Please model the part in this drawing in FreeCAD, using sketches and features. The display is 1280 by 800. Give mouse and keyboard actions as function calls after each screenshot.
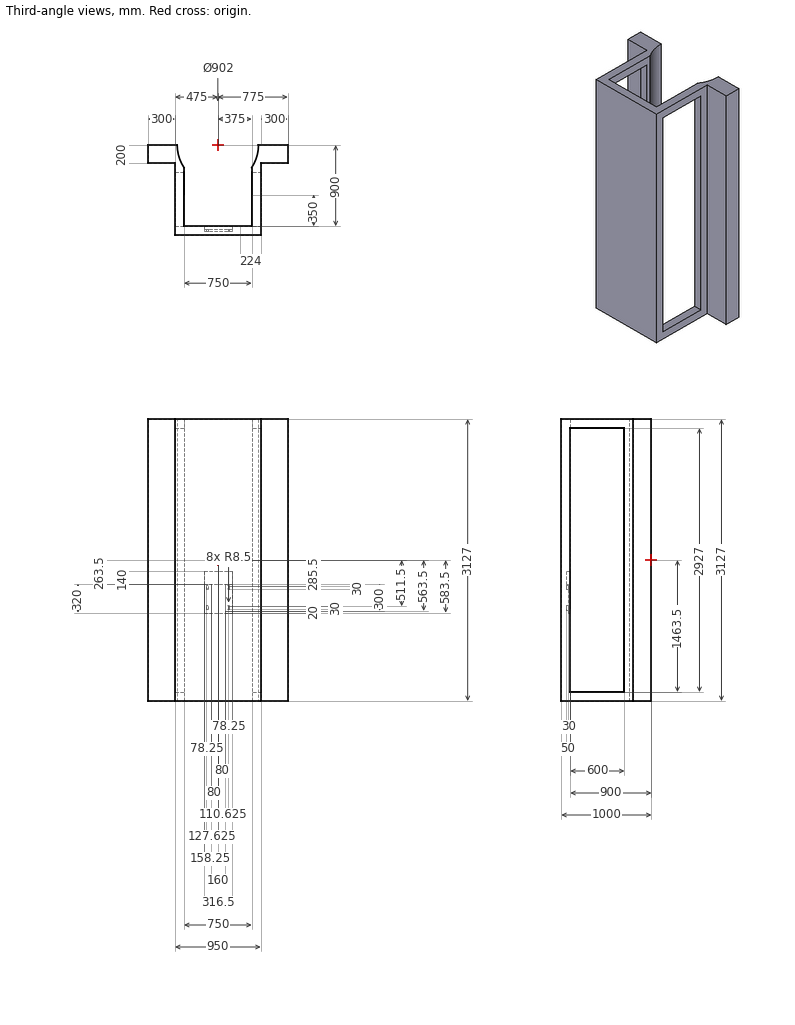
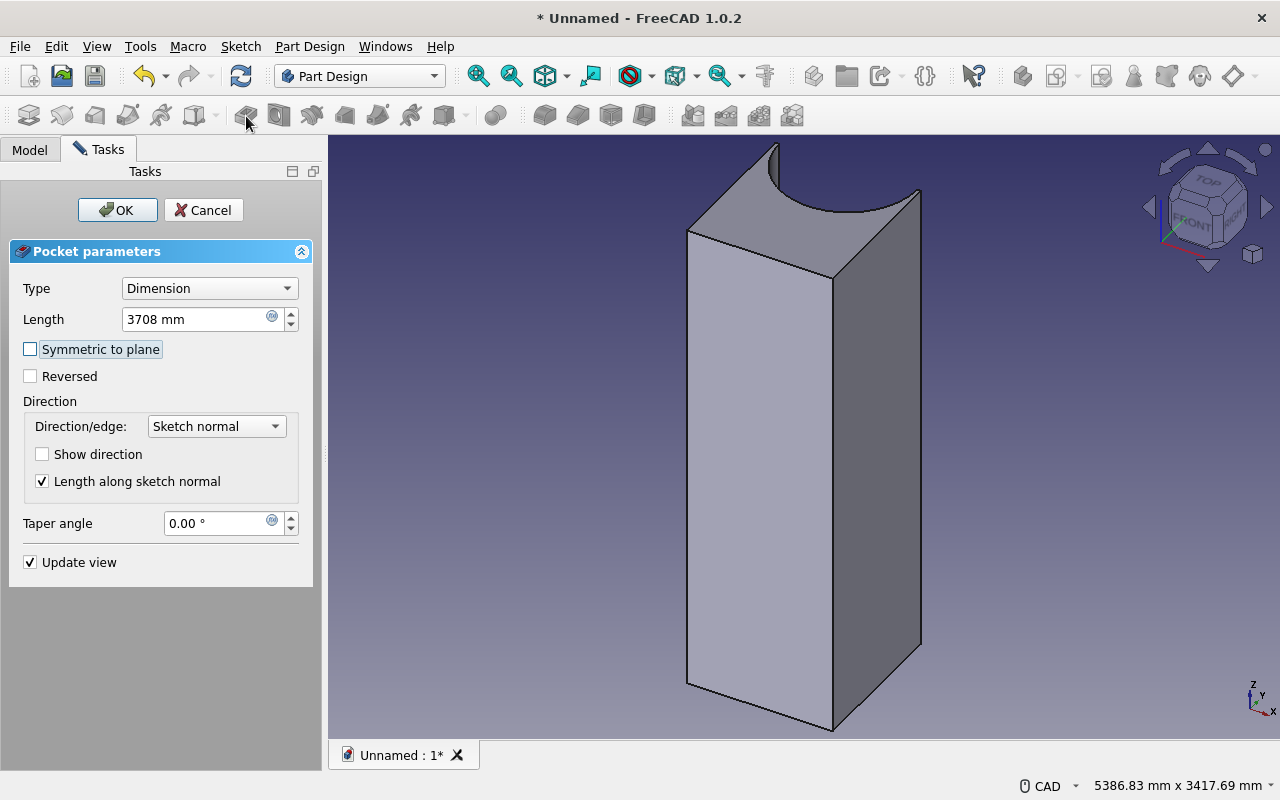
click(118, 210)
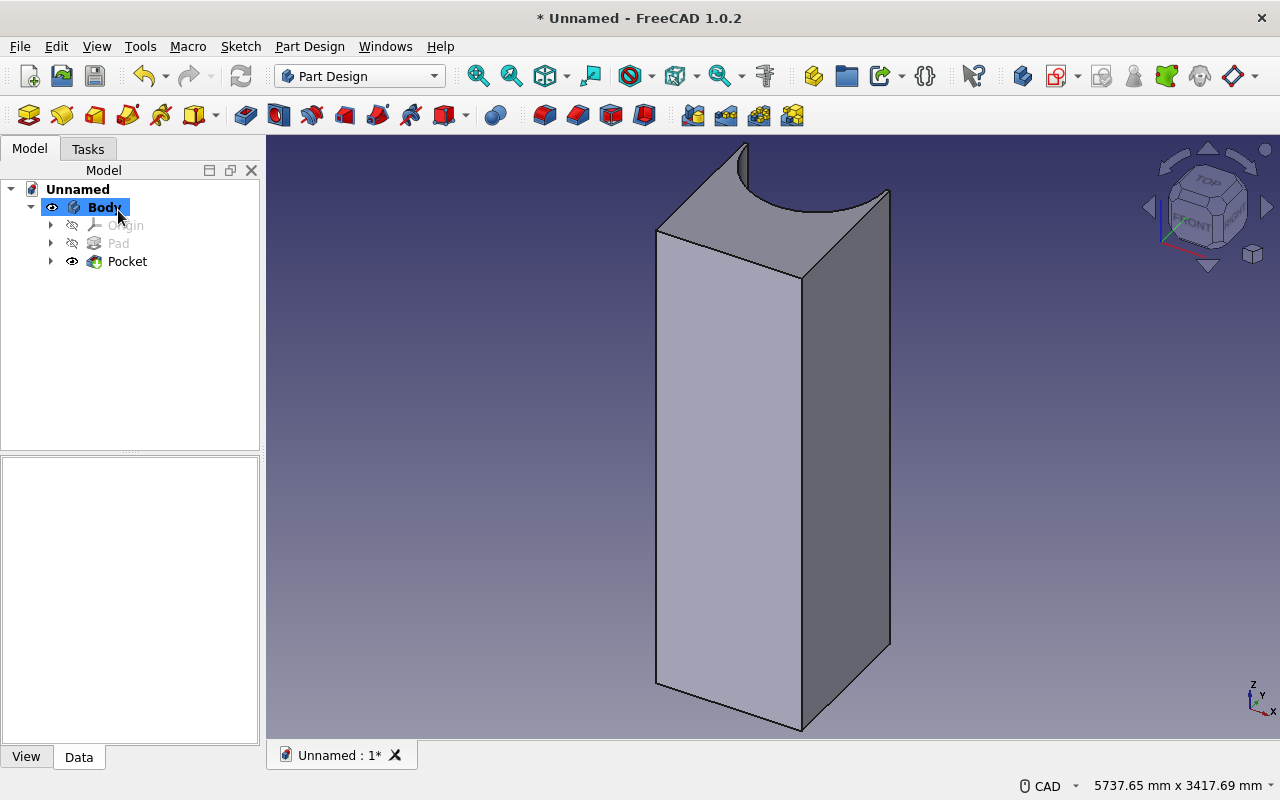
click(769, 242)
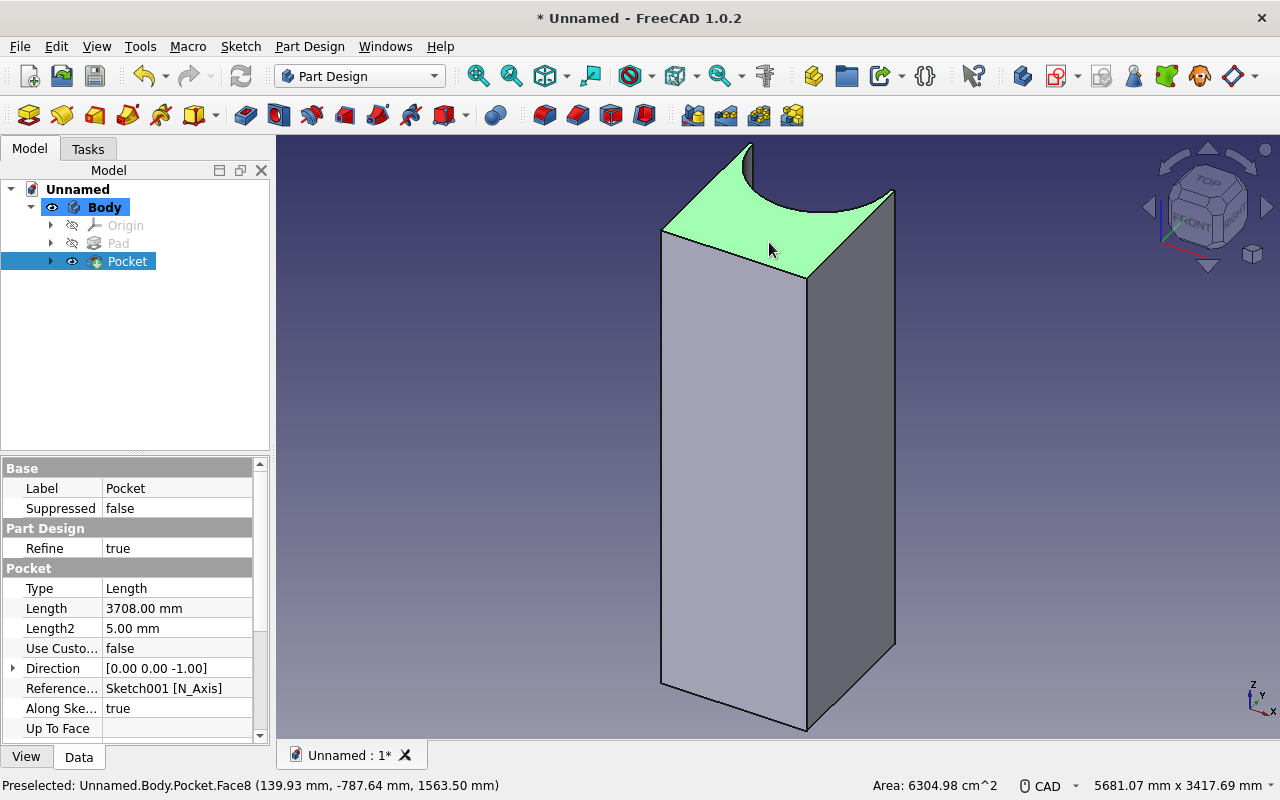
click(1056, 76)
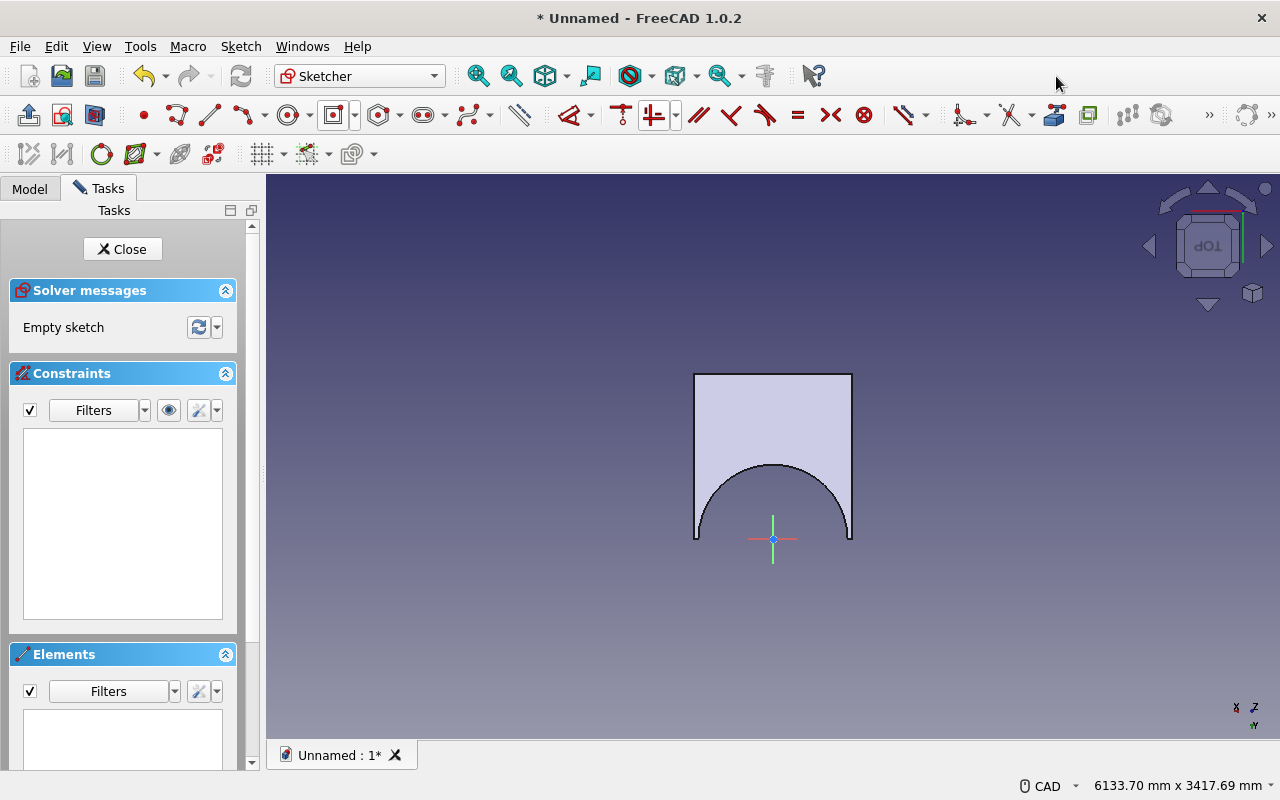
scroll(829, 577, up, 4)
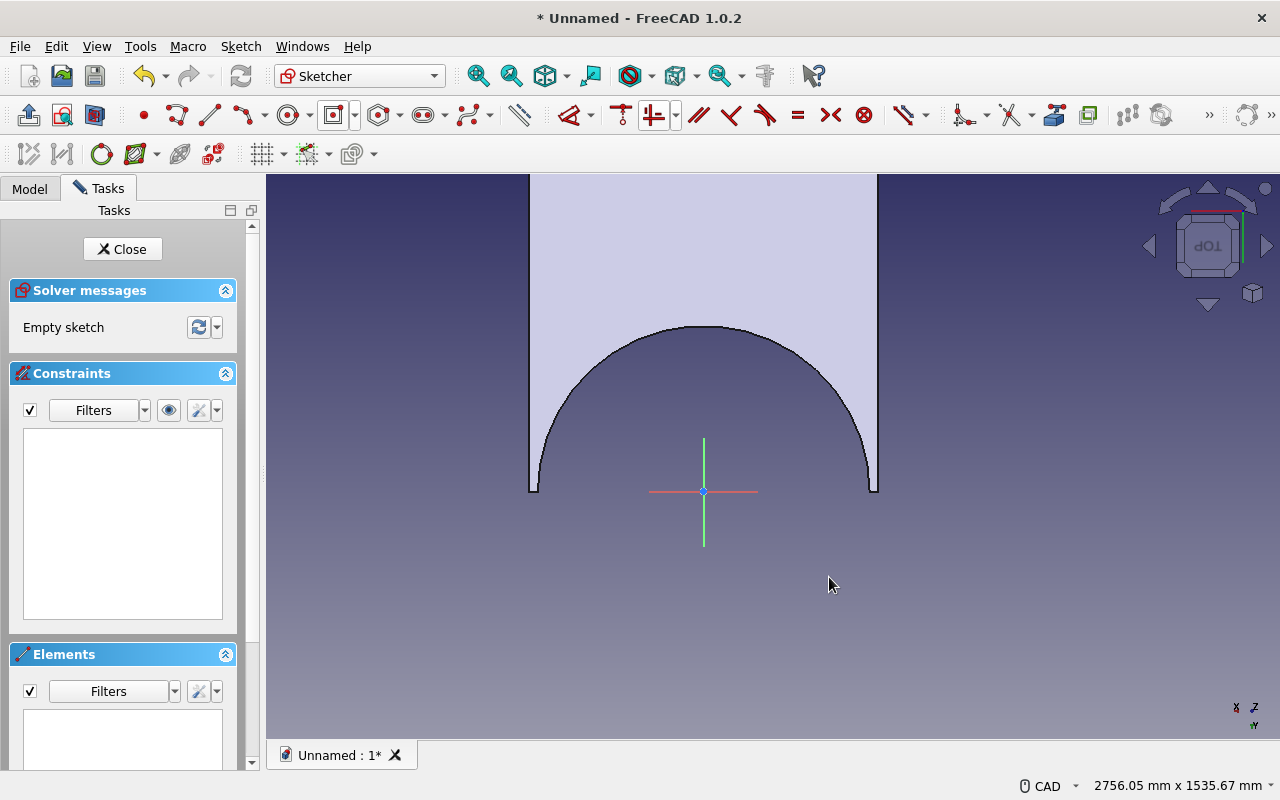
key(g)
key(r)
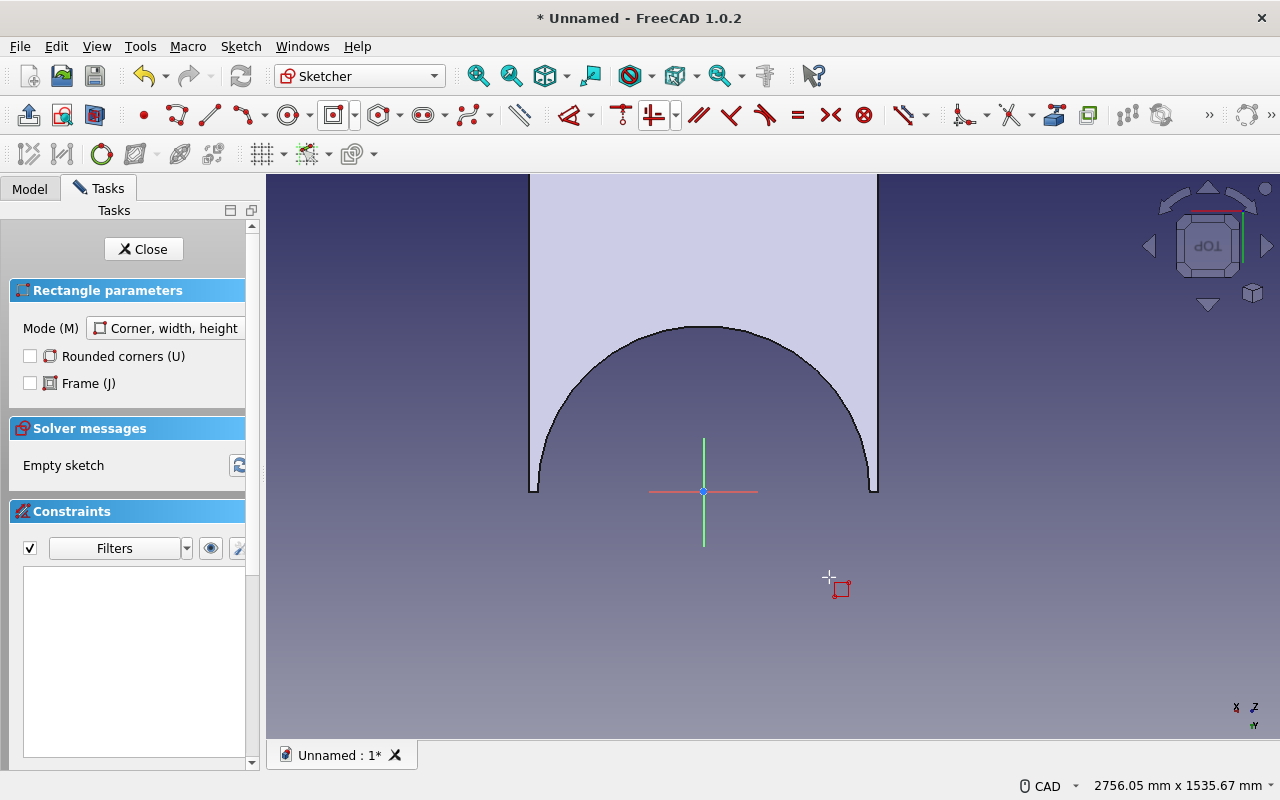
click(878, 418)
click(989, 492)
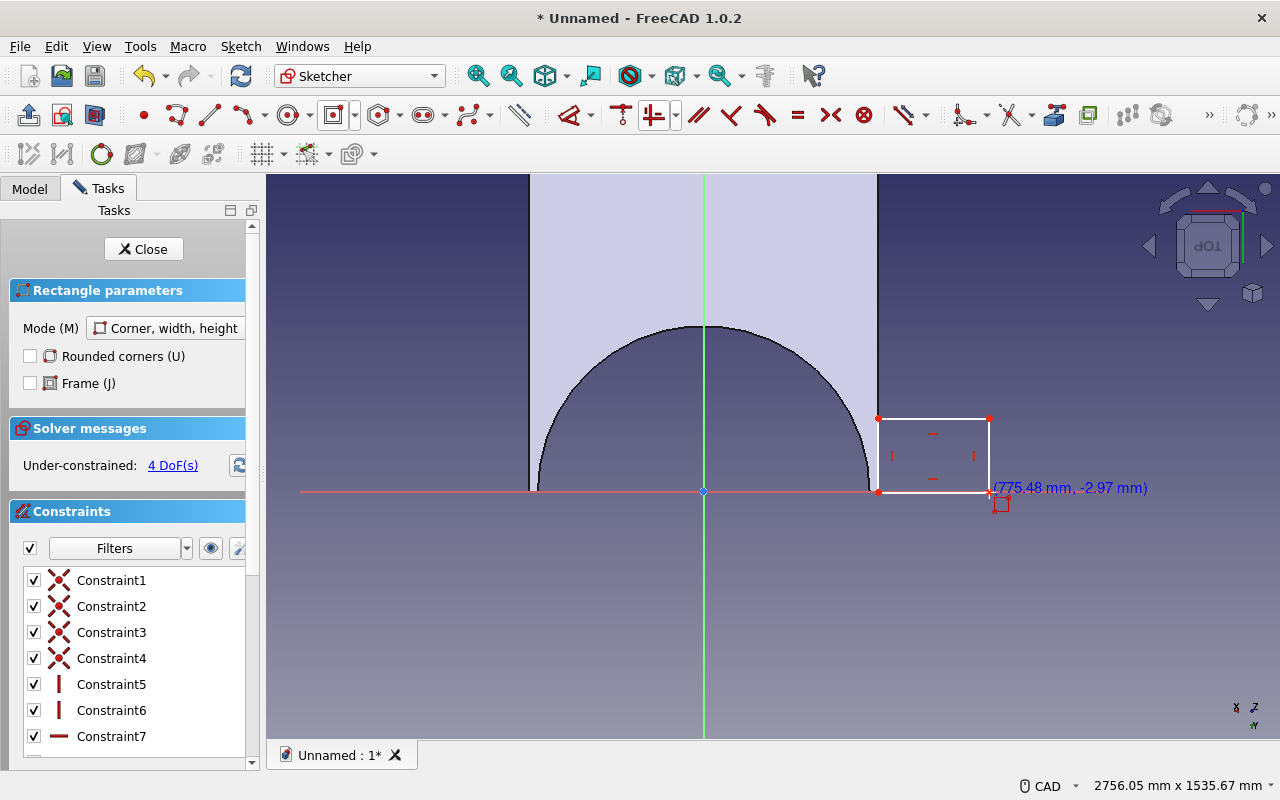
click(419, 418)
click(529, 492)
key(Escape)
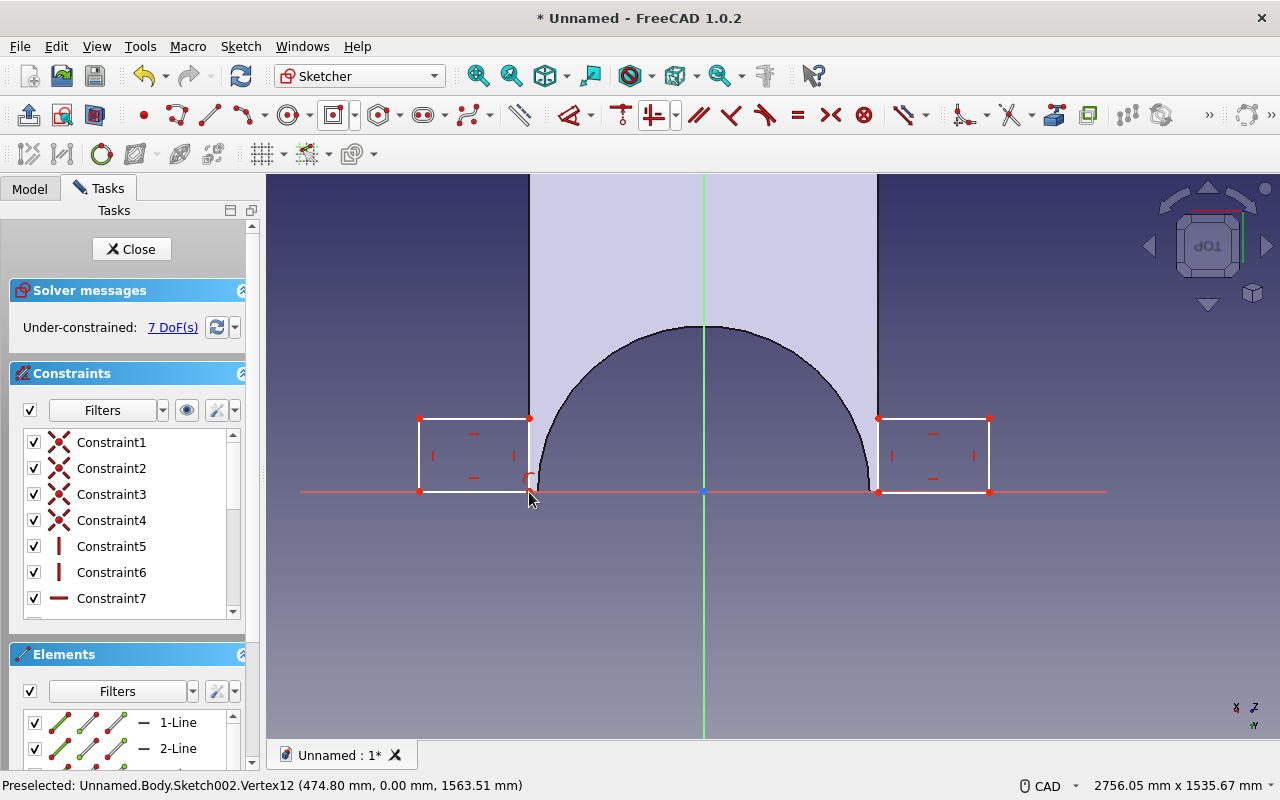
click(878, 493)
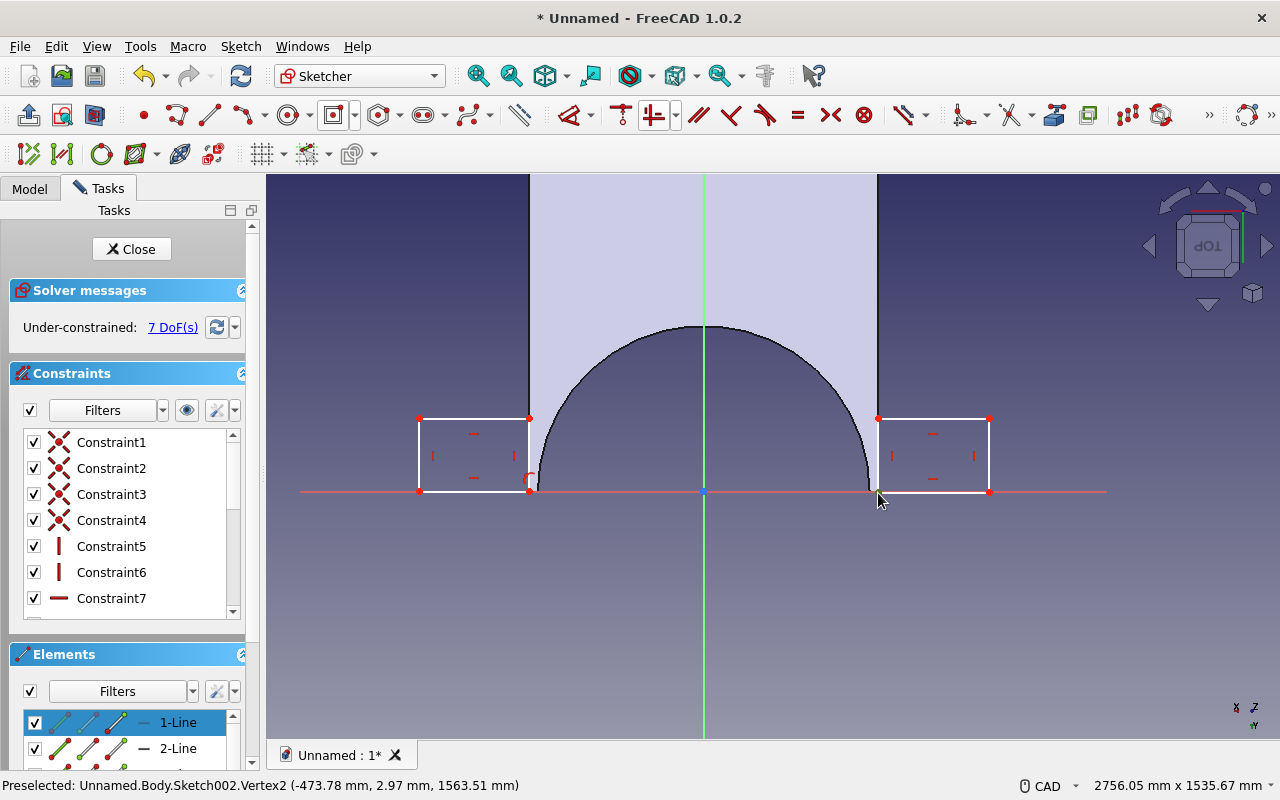
click(353, 492)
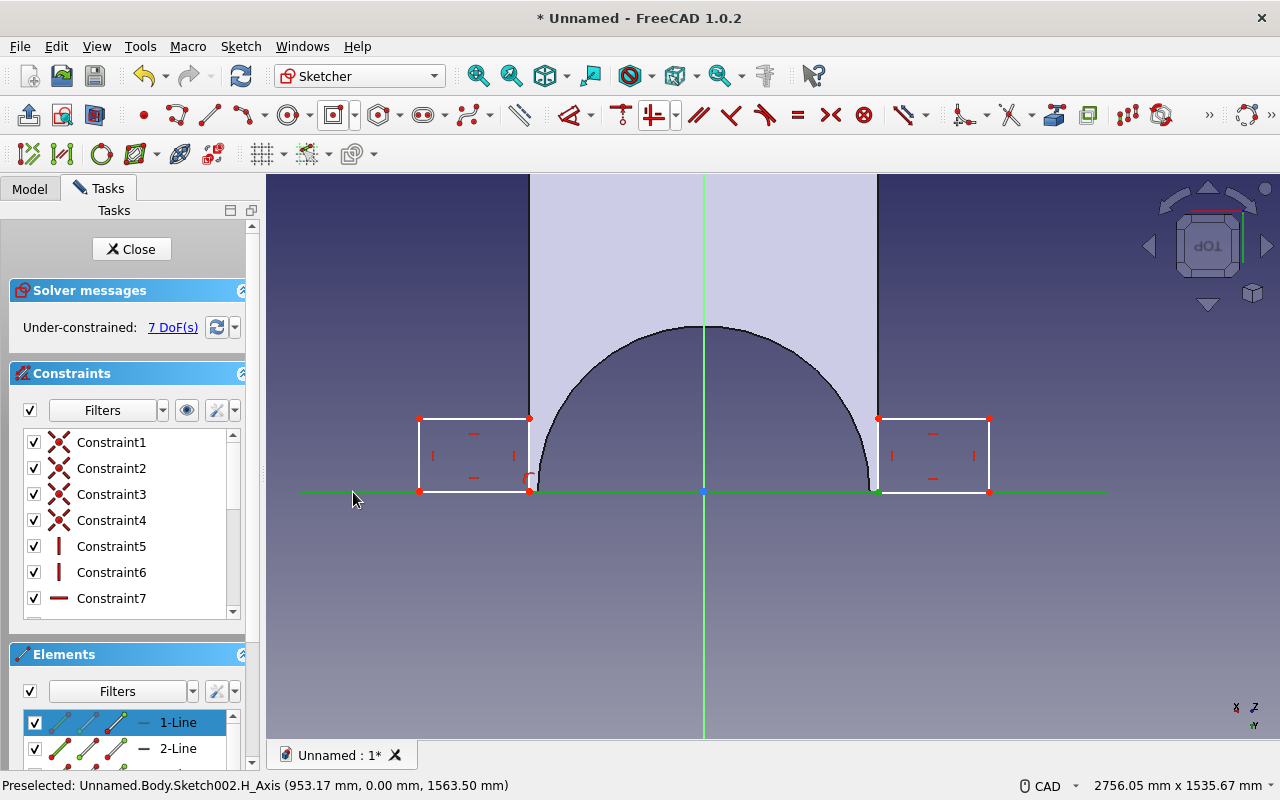
click(621, 116)